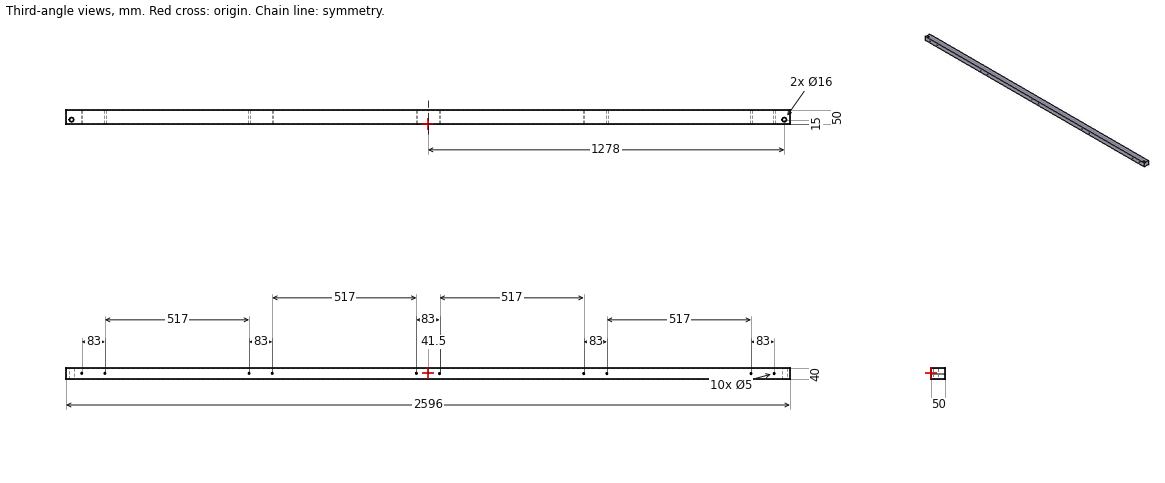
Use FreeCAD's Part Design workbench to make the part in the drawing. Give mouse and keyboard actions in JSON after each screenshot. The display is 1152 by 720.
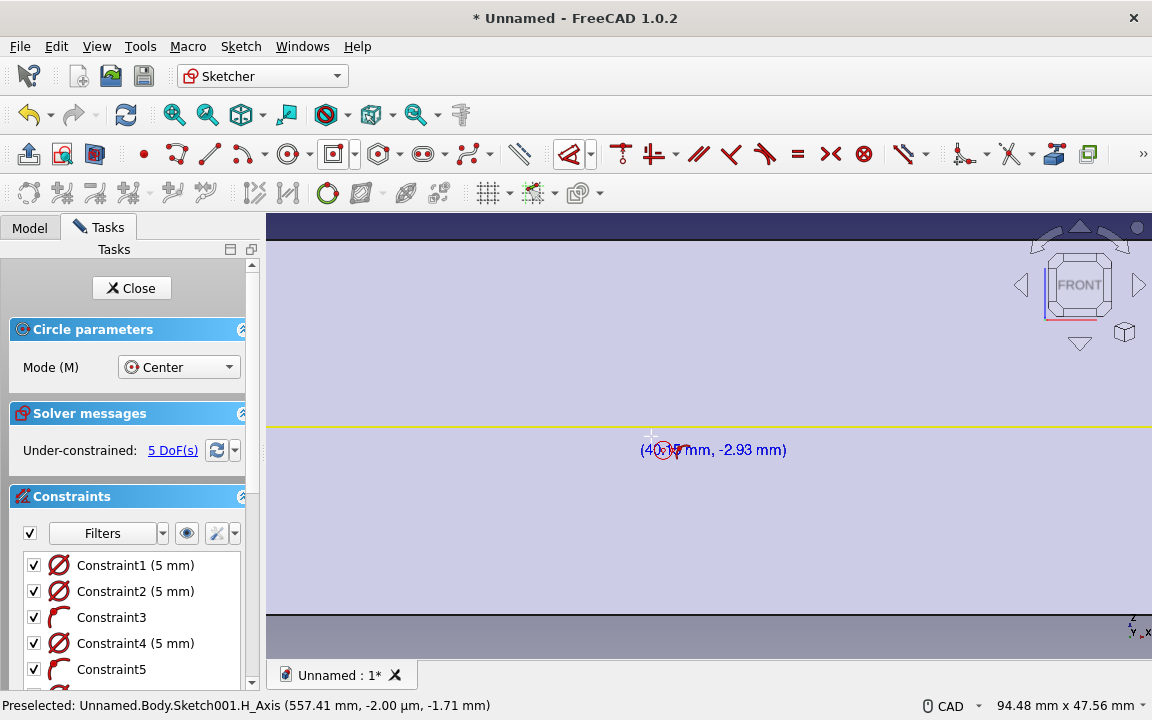
{"action": "scroll", "coordinate": [651, 436], "scroll_direction": "down", "scroll_amount": 18}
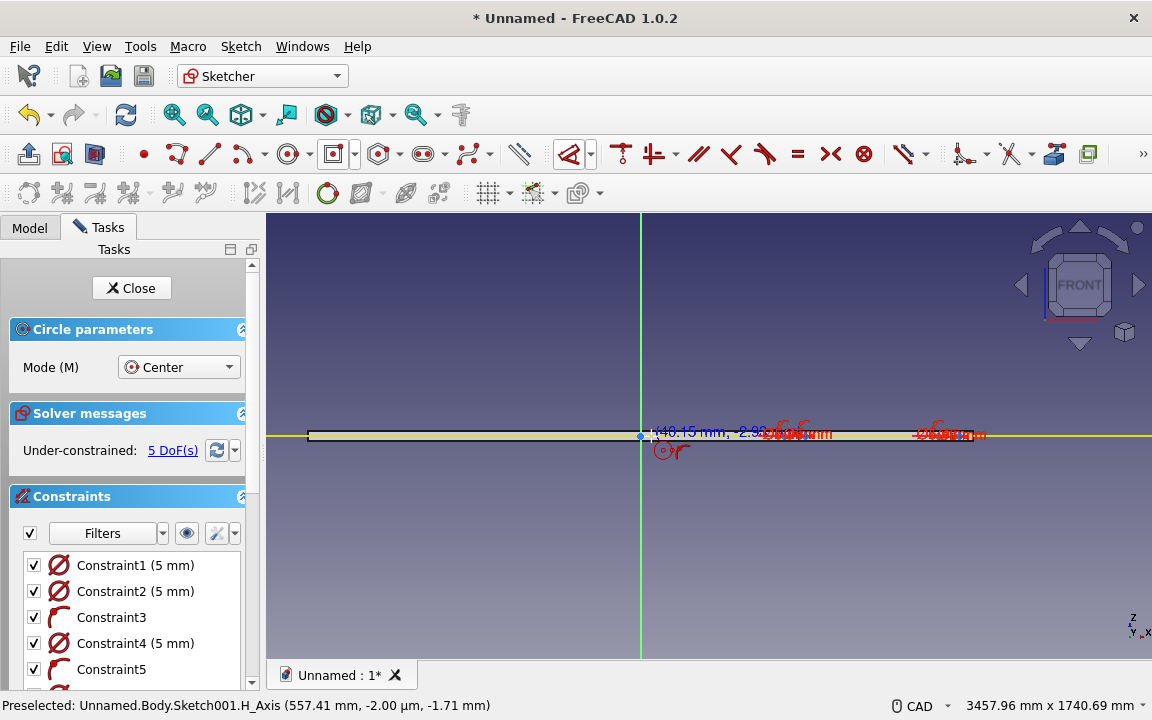
{"action": "scroll", "coordinate": [651, 436], "scroll_direction": "up", "scroll_amount": 3}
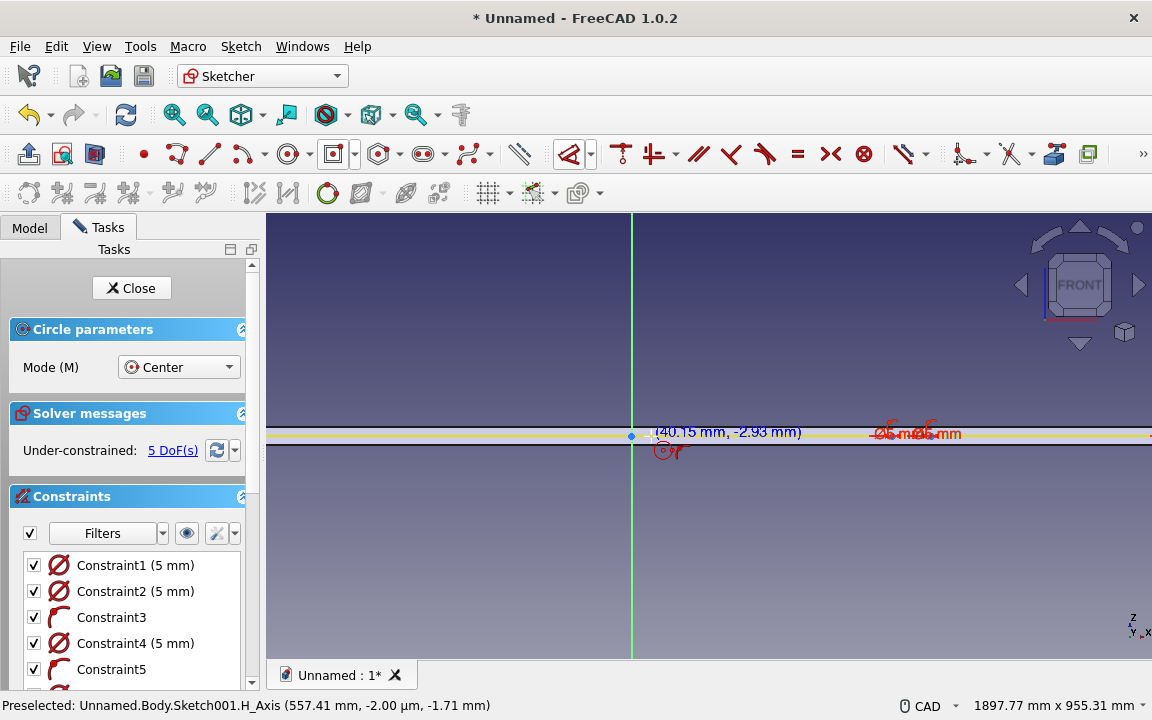
{"action": "left_click", "coordinate": [651, 436]}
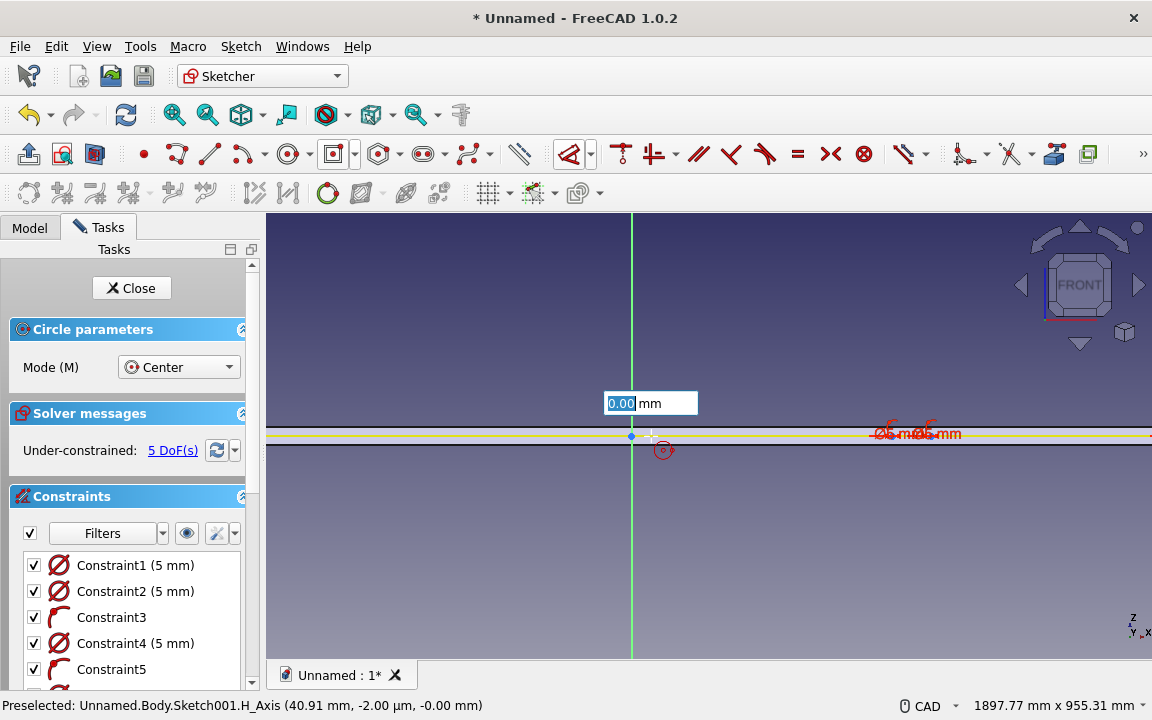
{"action": "scroll", "coordinate": [651, 437], "scroll_direction": "up", "scroll_amount": 14}
{"action": "mouse_move", "coordinate": [642, 432]}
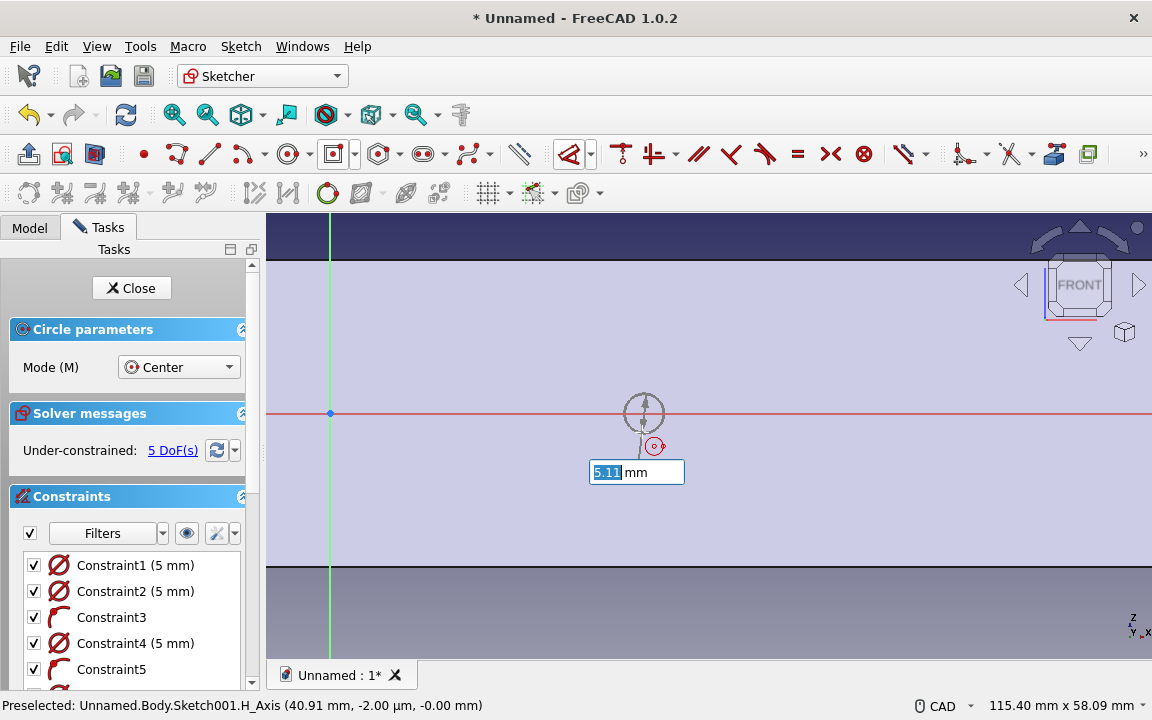
{"action": "type", "text": "5"}
{"action": "key", "text": "Return"}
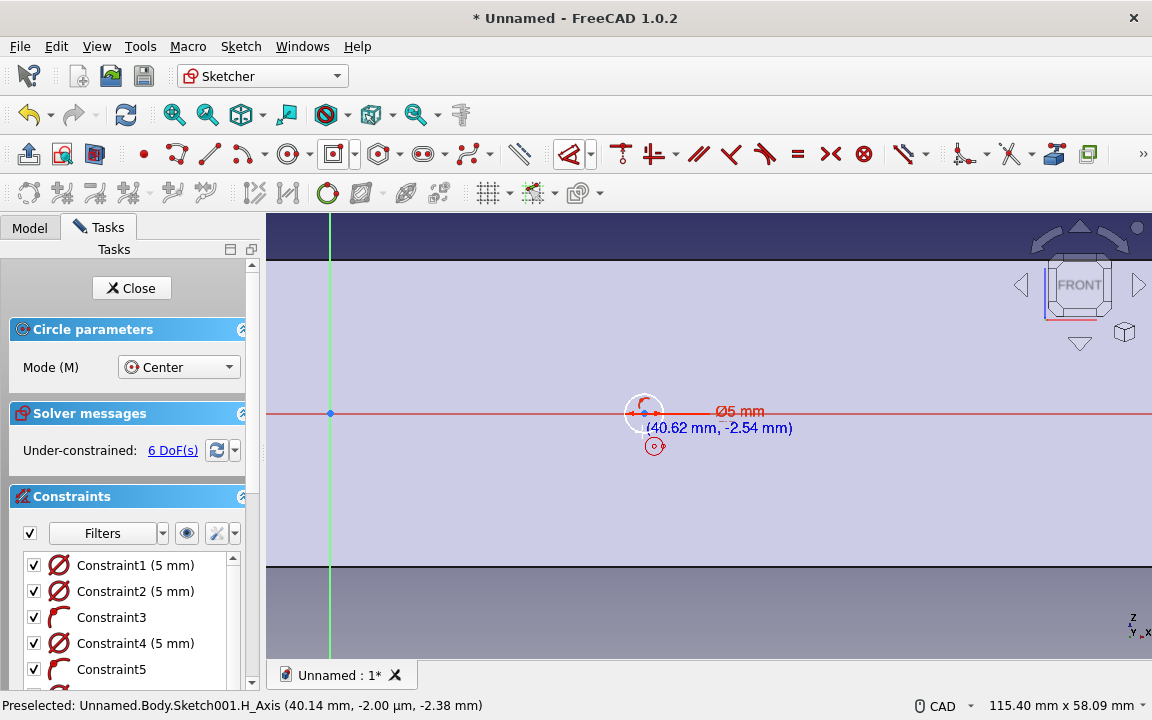
{"action": "scroll", "coordinate": [651, 437], "scroll_direction": "down", "scroll_amount": 17}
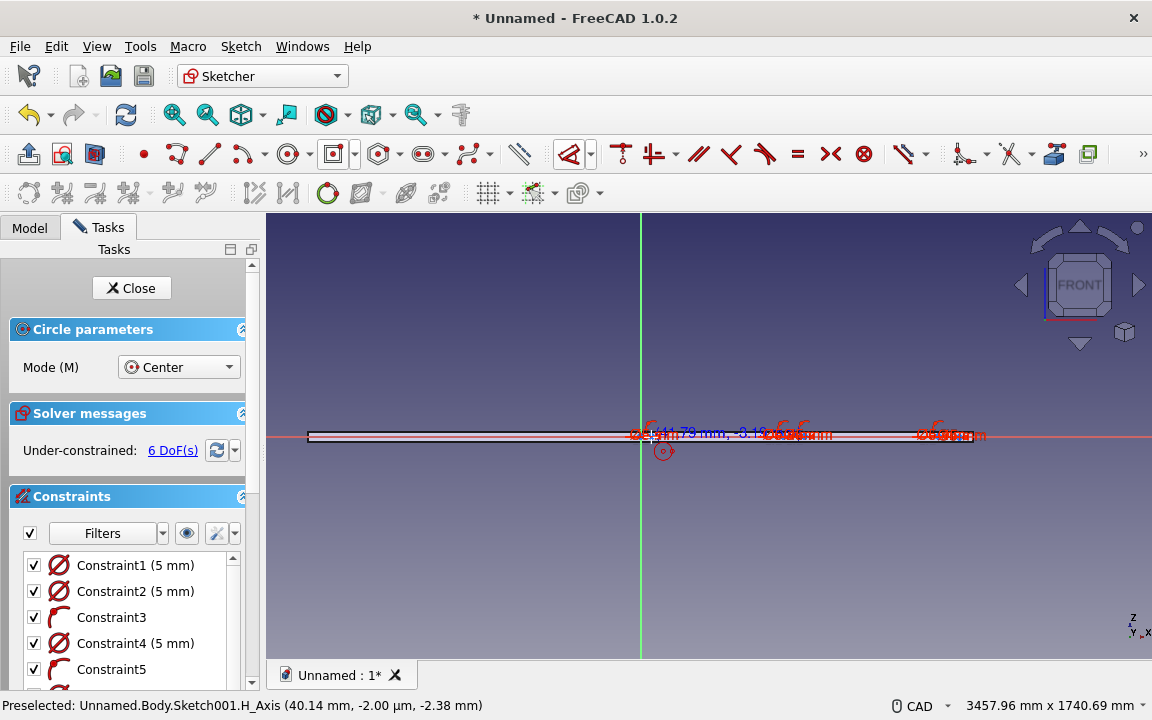
{"action": "scroll", "coordinate": [630, 437], "scroll_direction": "up", "scroll_amount": 18}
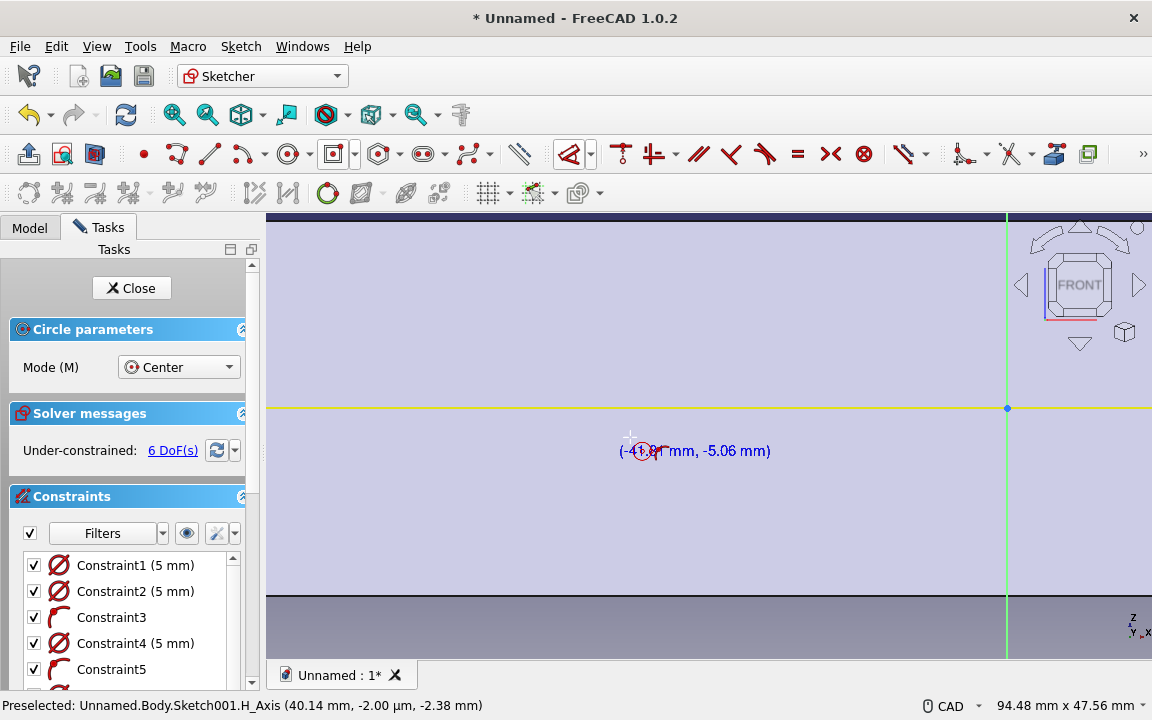
{"action": "scroll", "coordinate": [630, 437], "scroll_direction": "down", "scroll_amount": 18}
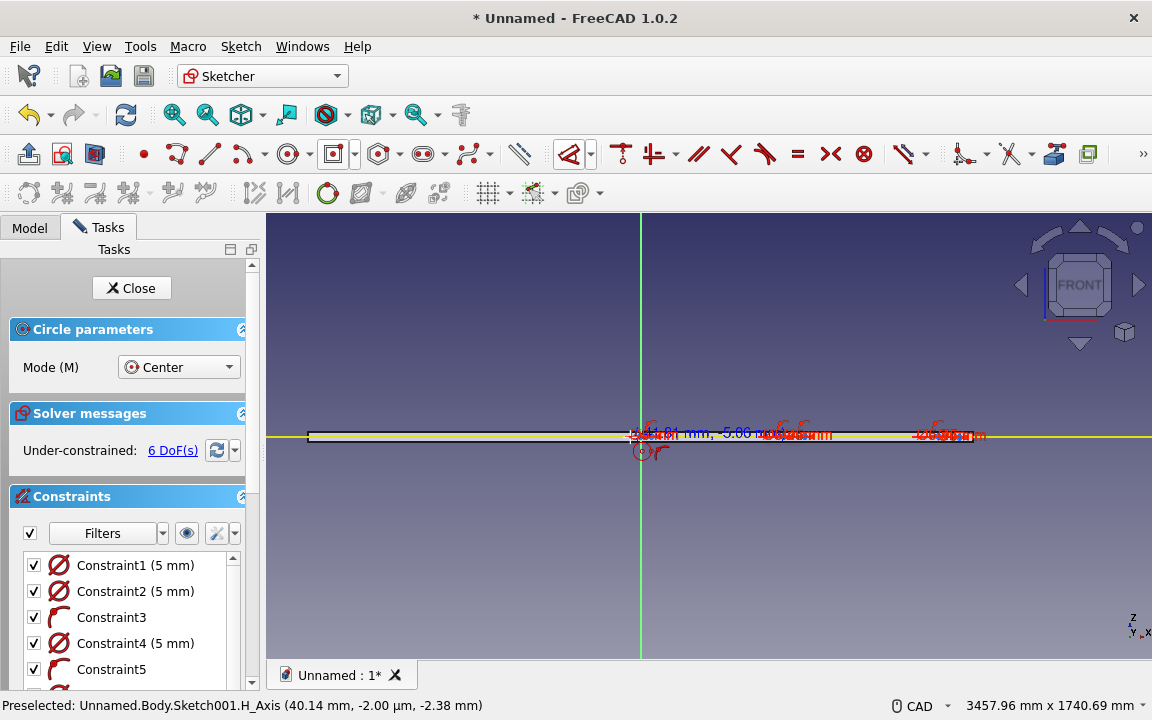
{"action": "scroll", "coordinate": [630, 437], "scroll_direction": "up", "scroll_amount": 3}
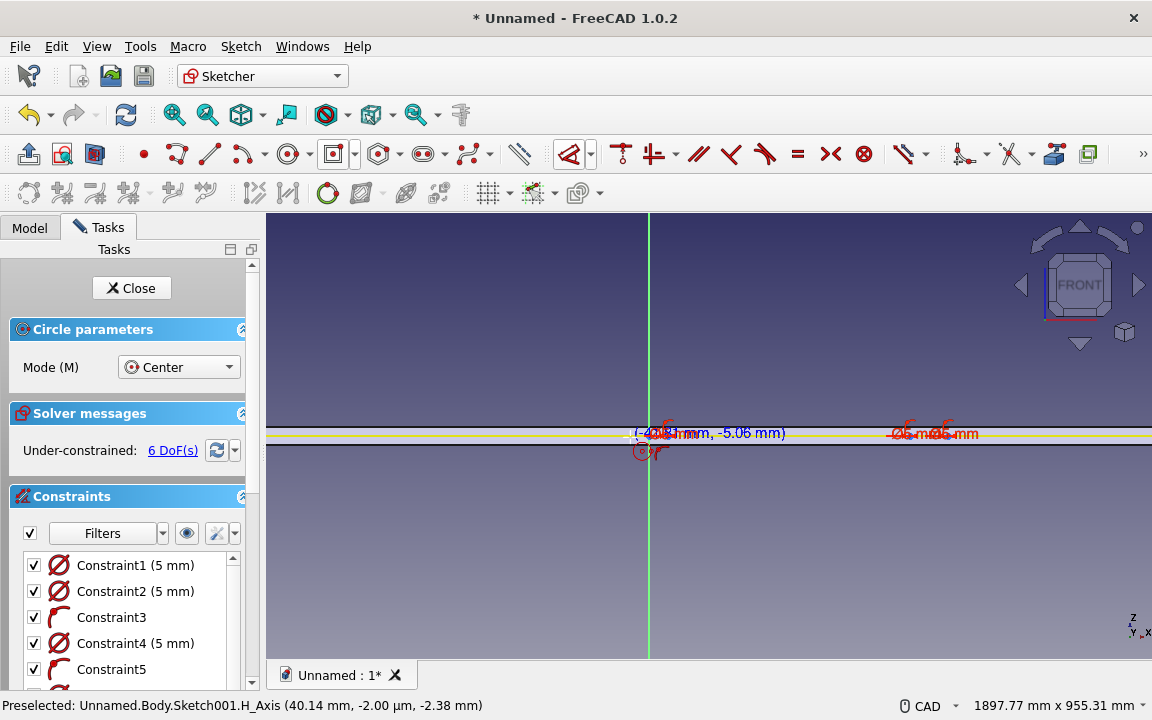
{"action": "left_click", "coordinate": [630, 436]}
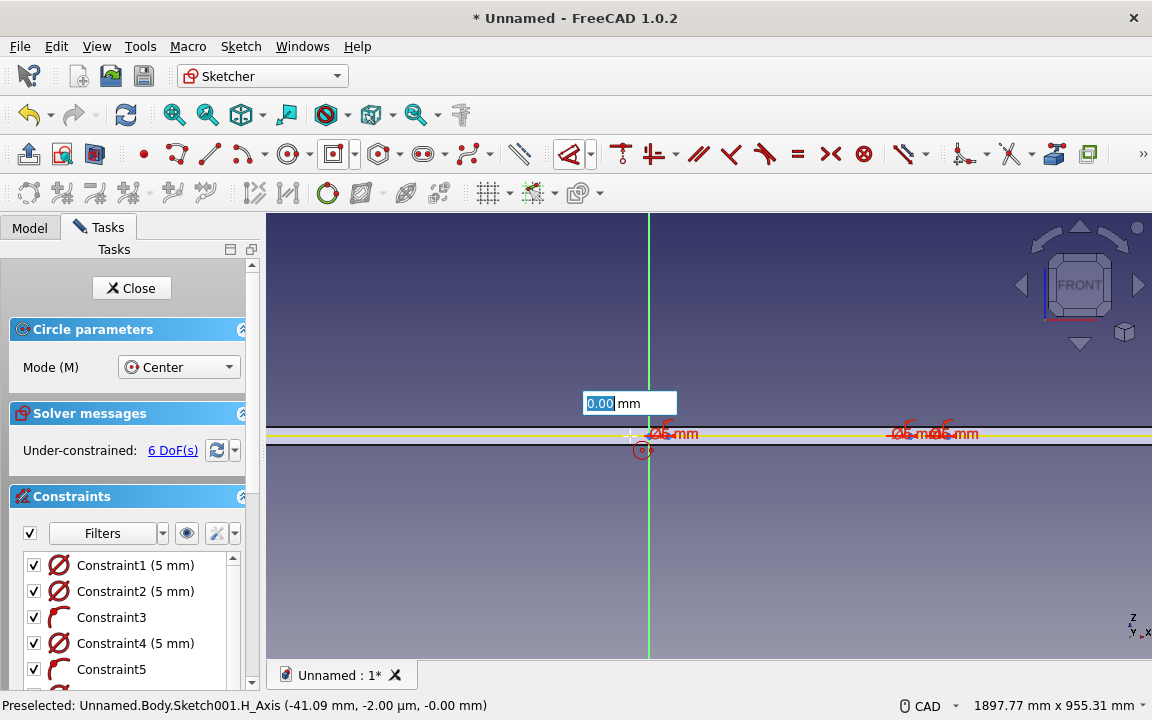
{"action": "scroll", "coordinate": [629, 437], "scroll_direction": "up", "scroll_amount": 14}
{"action": "mouse_move", "coordinate": [629, 432]}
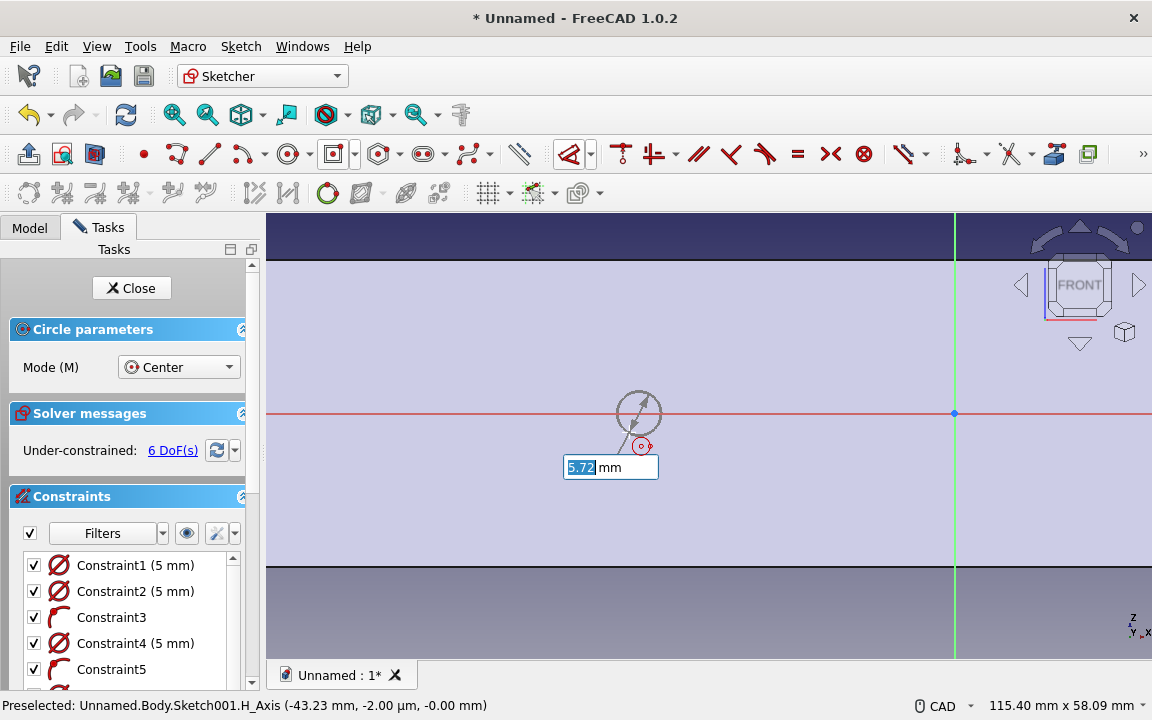
{"action": "type", "text": "5"}
{"action": "key", "text": "Return"}